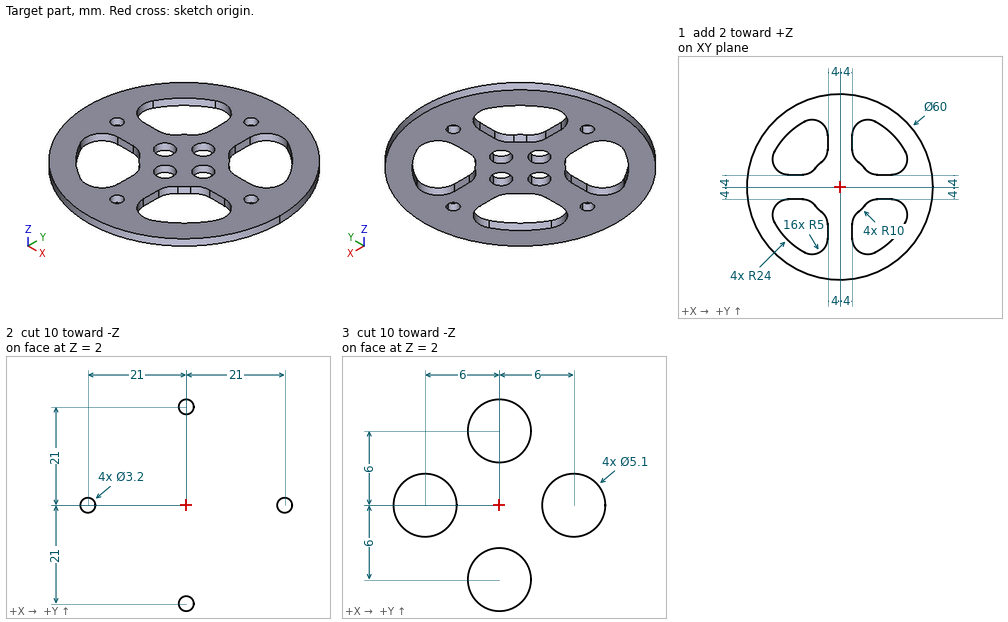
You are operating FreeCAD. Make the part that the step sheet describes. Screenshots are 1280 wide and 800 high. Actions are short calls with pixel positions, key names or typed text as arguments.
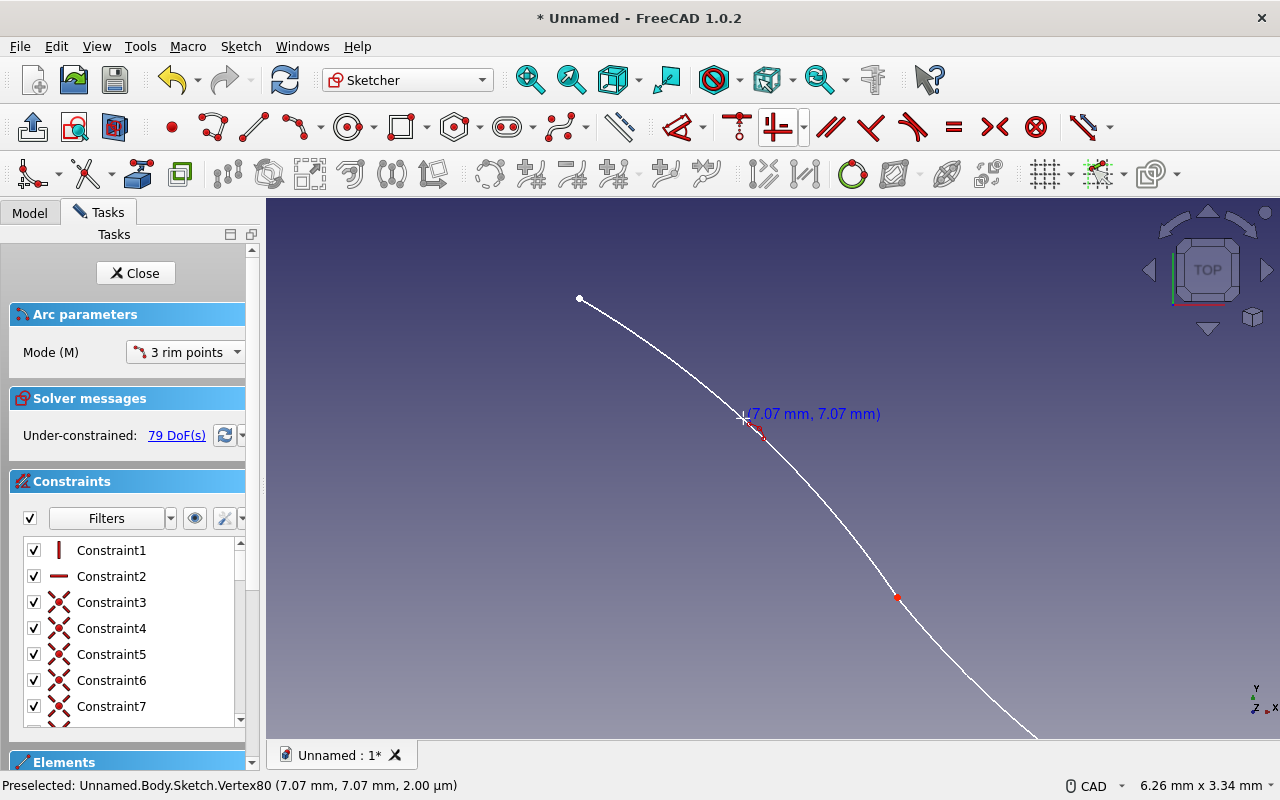
scroll(752, 422, down, 16)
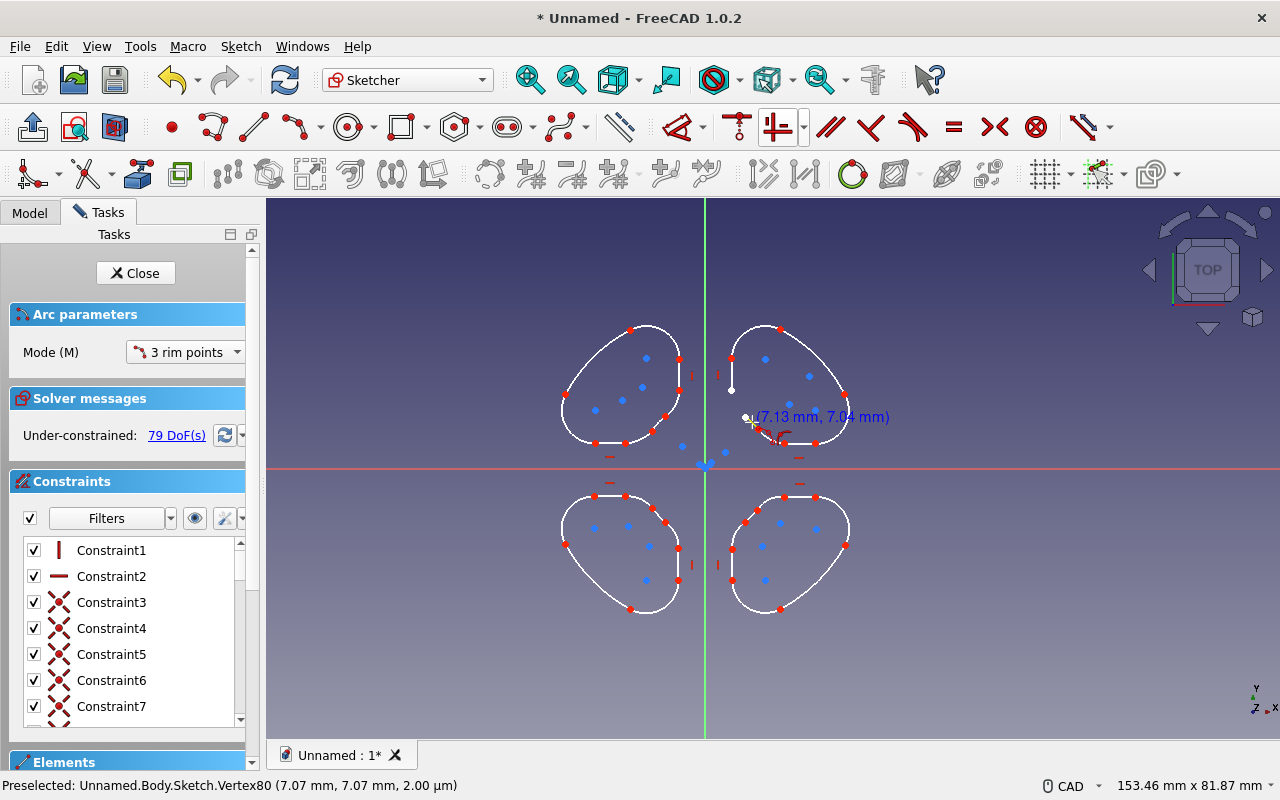
click(745, 417)
click(732, 390)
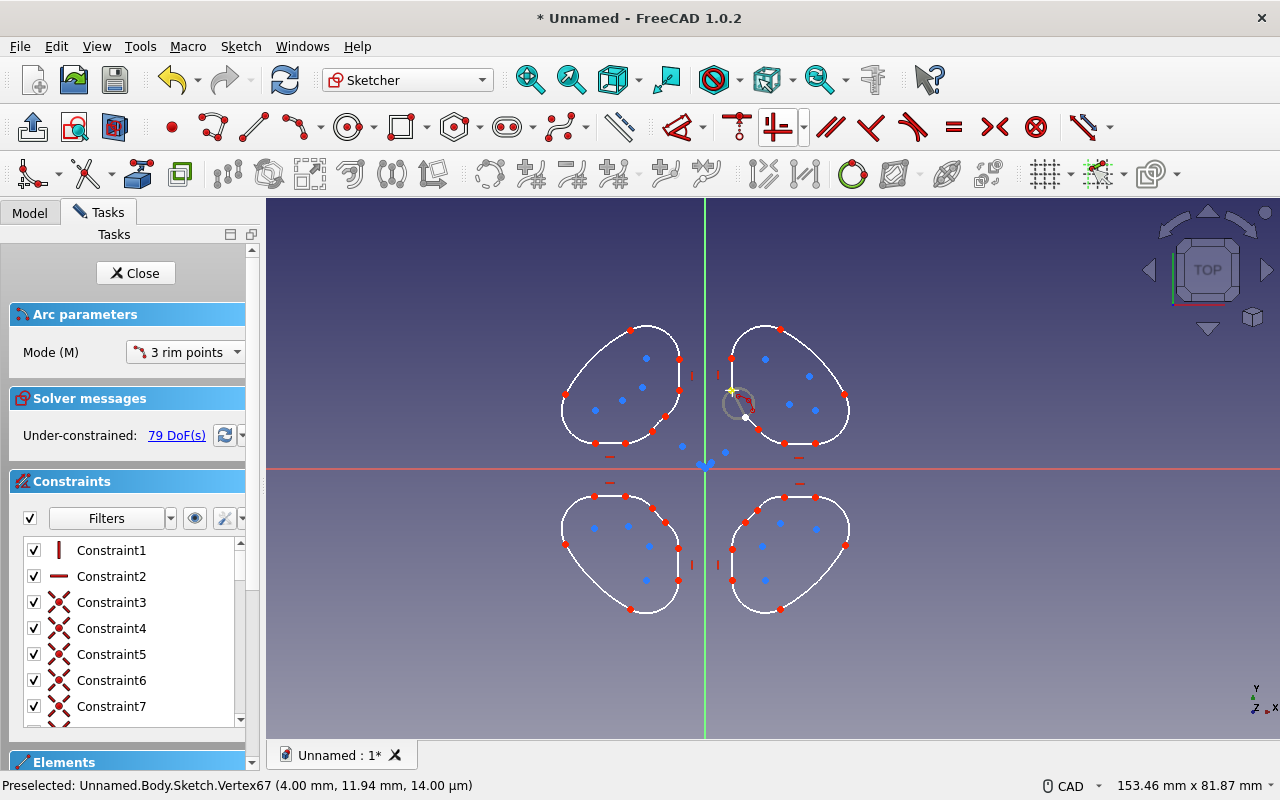
scroll(735, 404, up, 8)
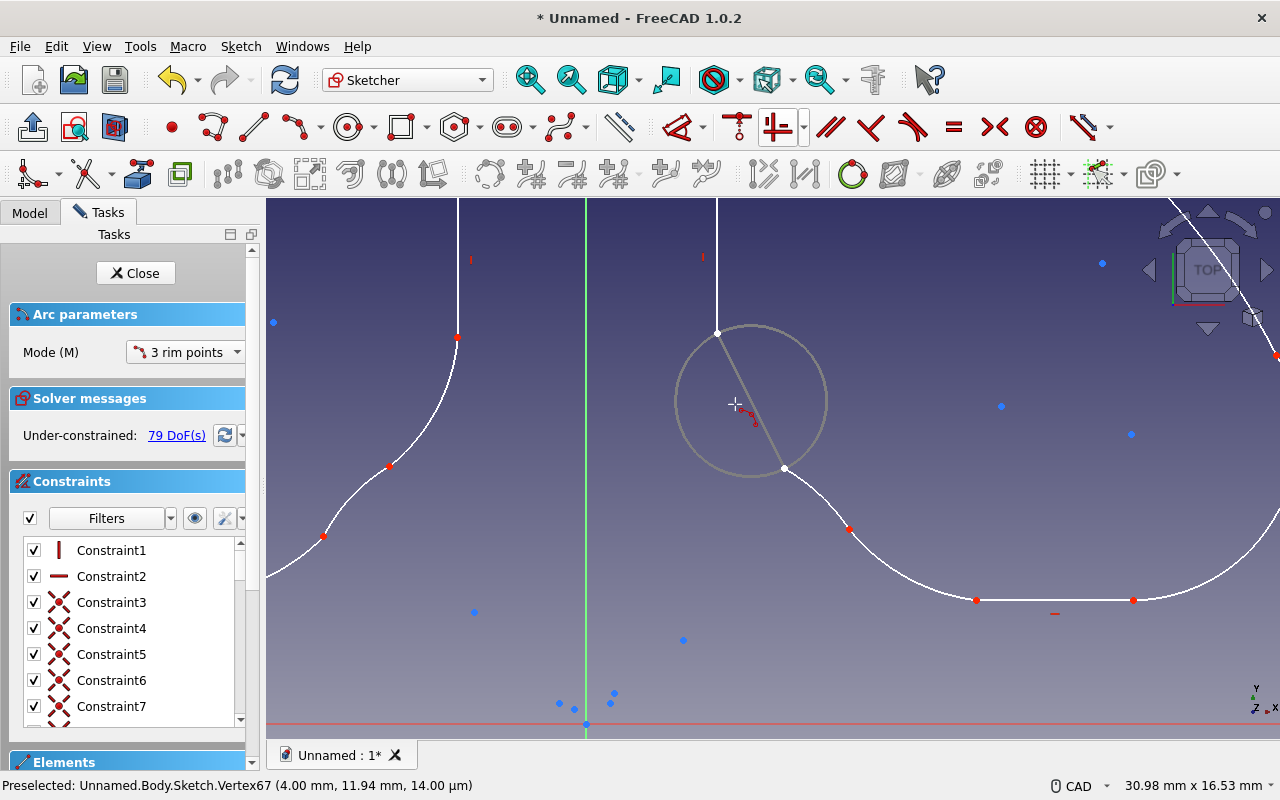
click(735, 405)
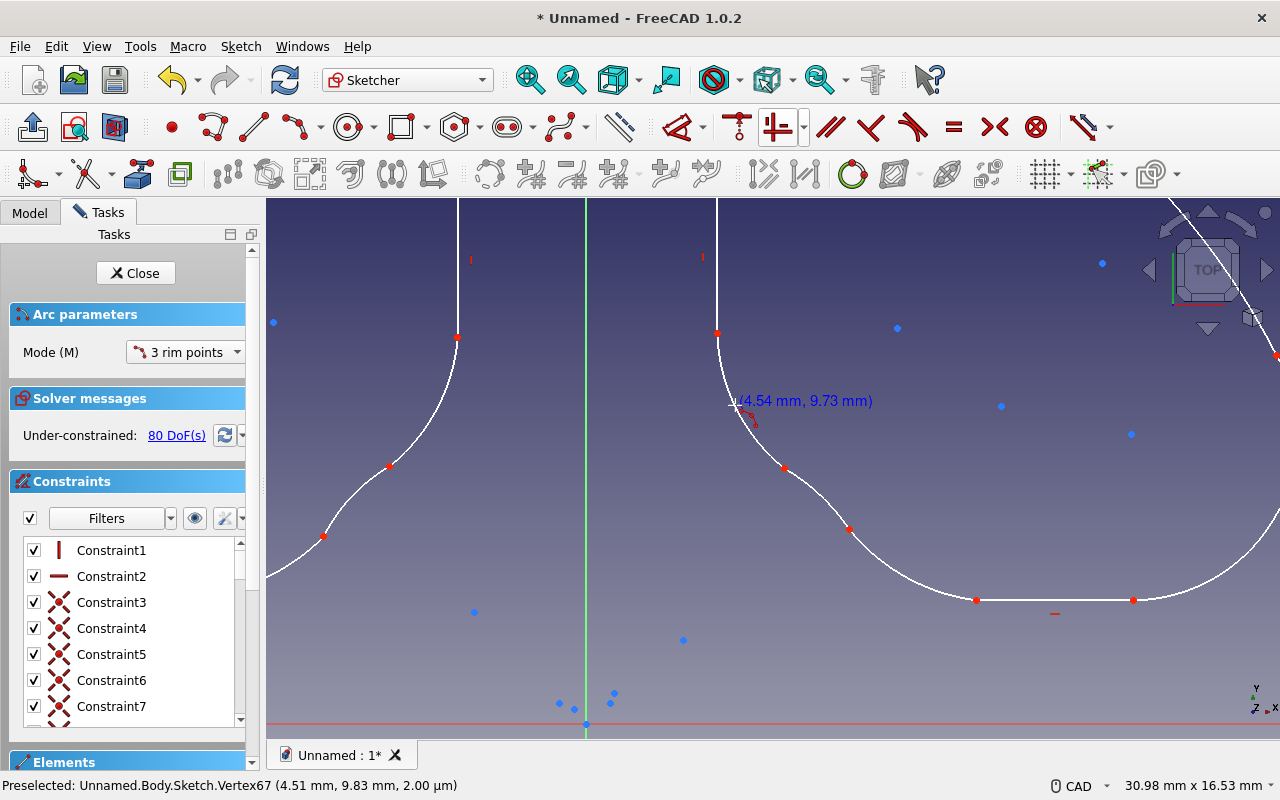
click(348, 128)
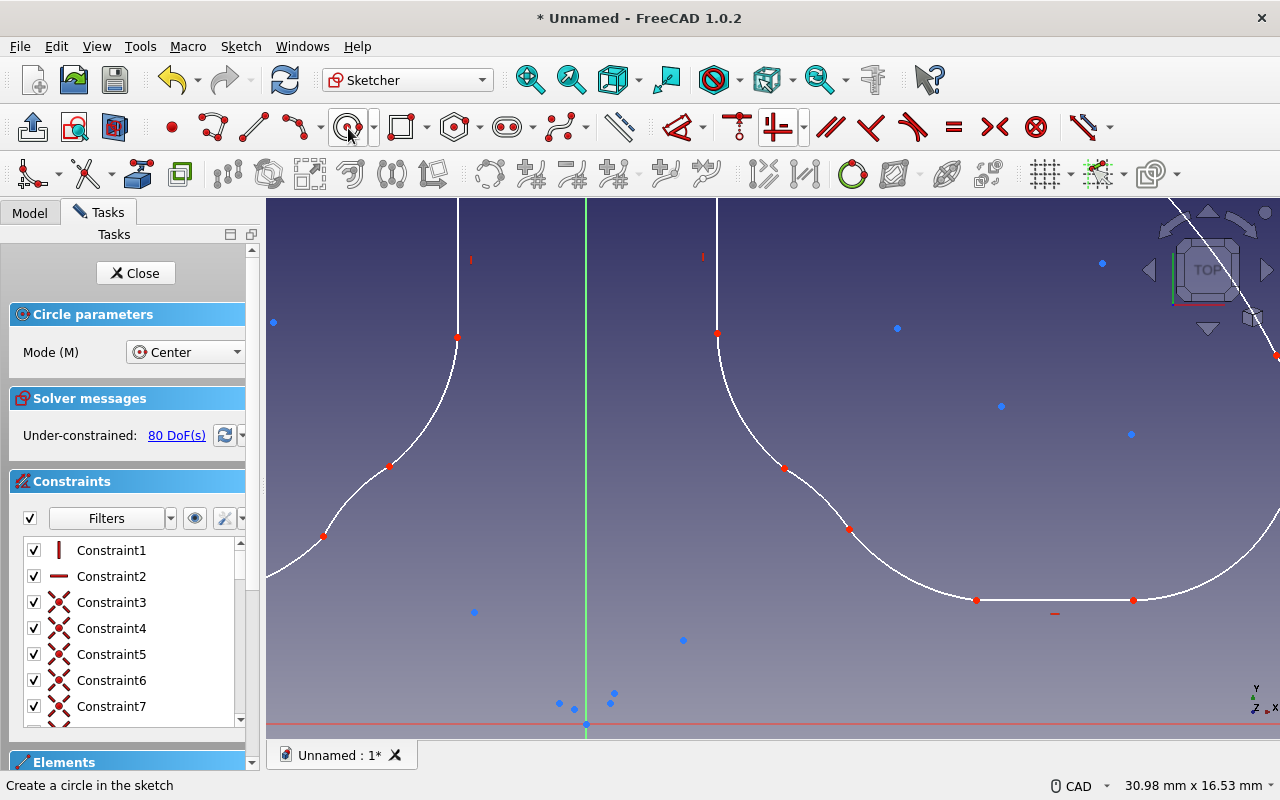
scroll(728, 418, down, 9)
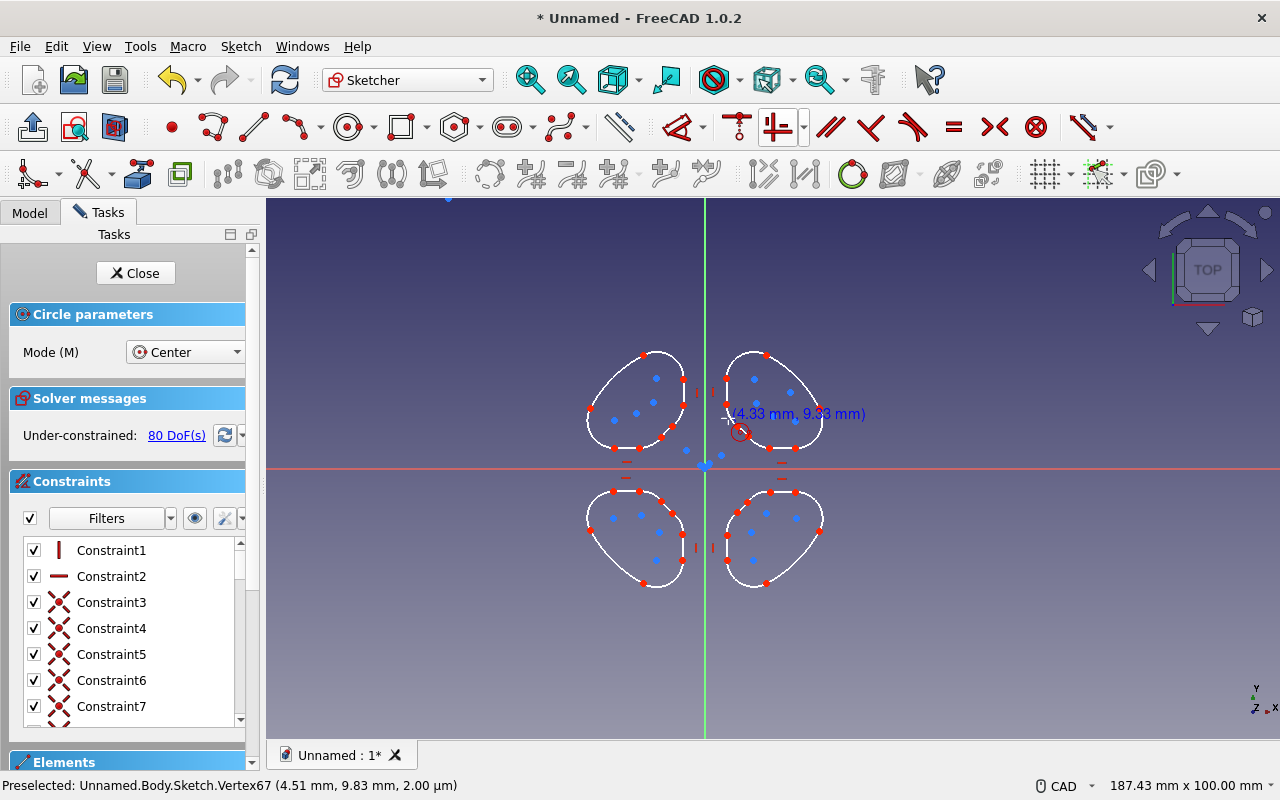
click(705, 469)
move(820, 354)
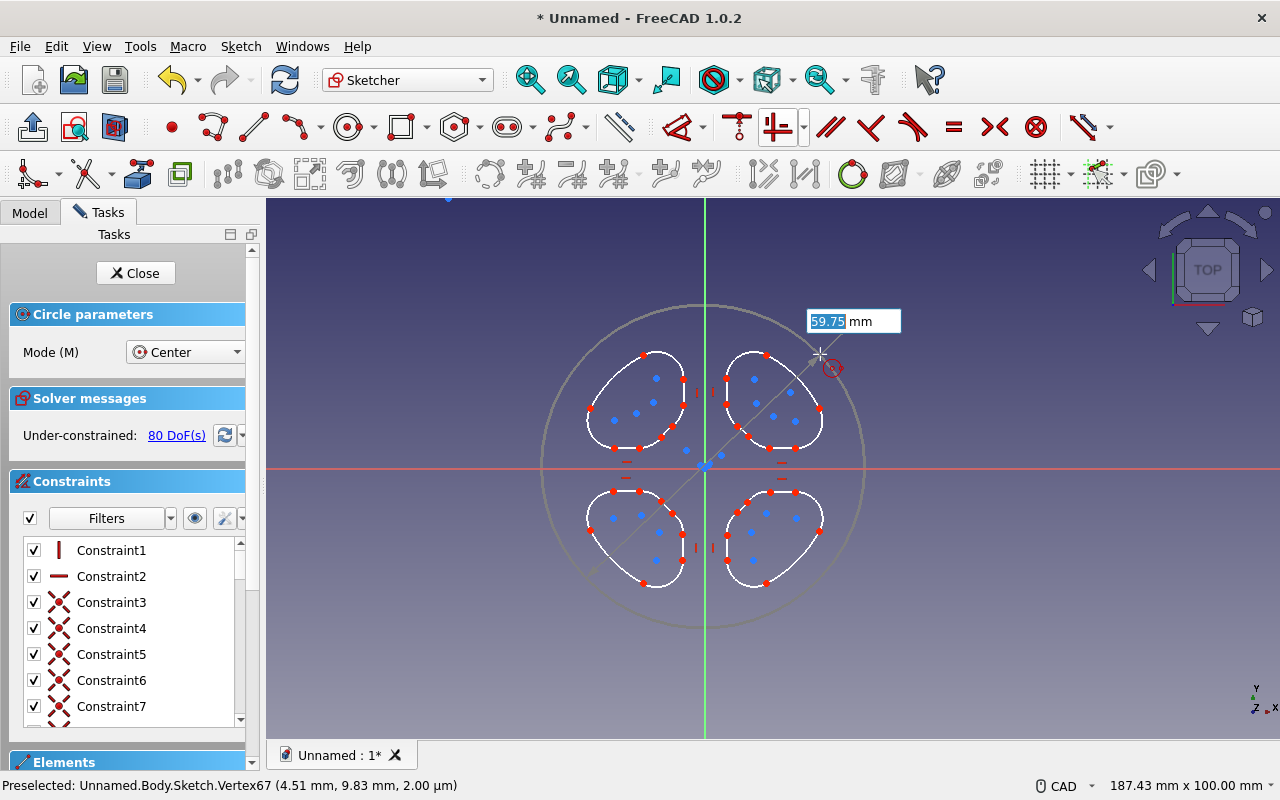
text(60)
key(Return)
key(Escape)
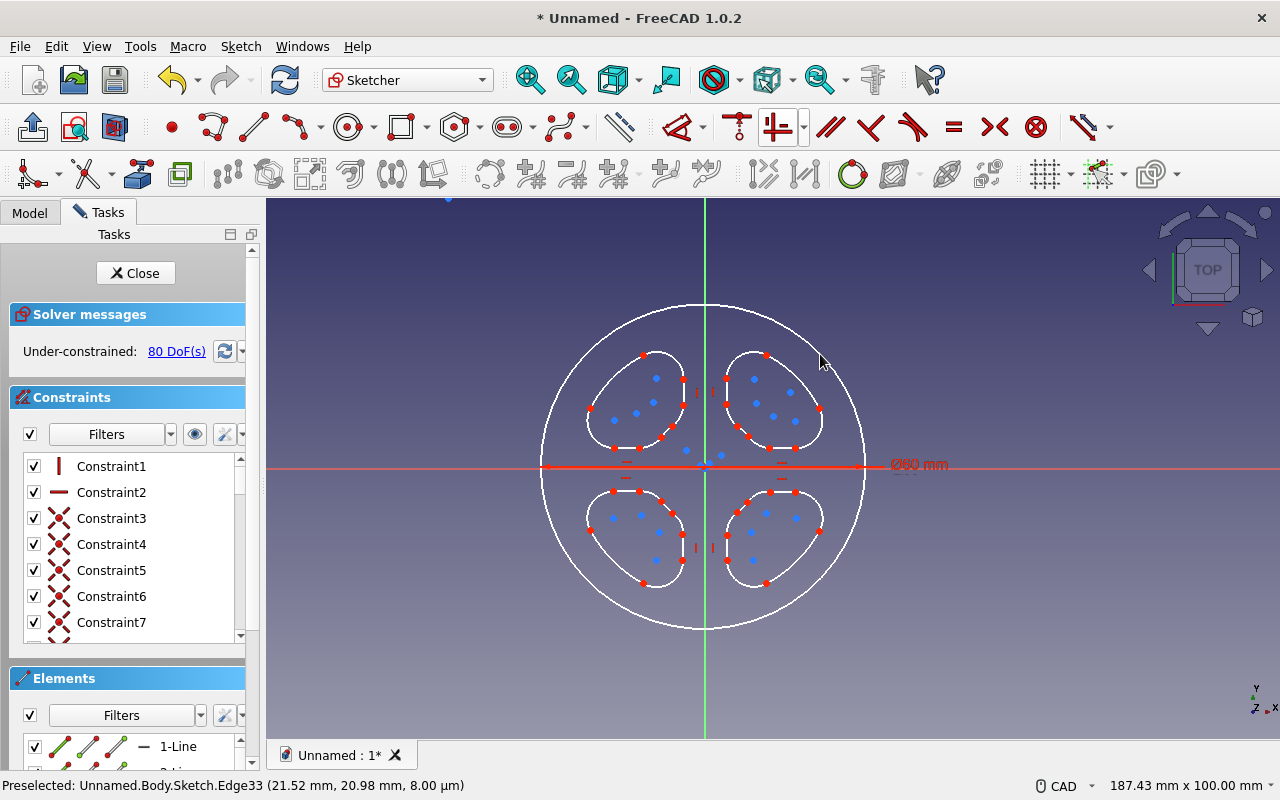
scroll(683, 545, up, 2)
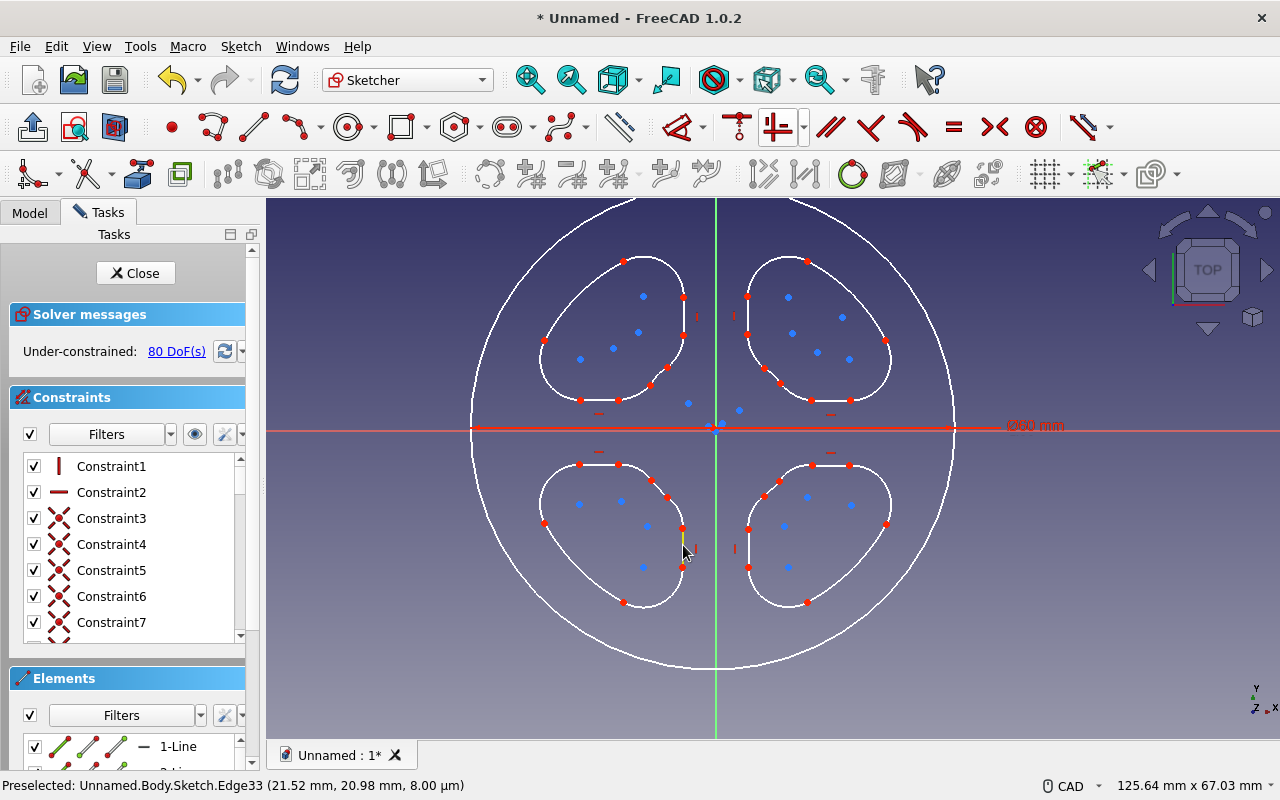
click(683, 544)